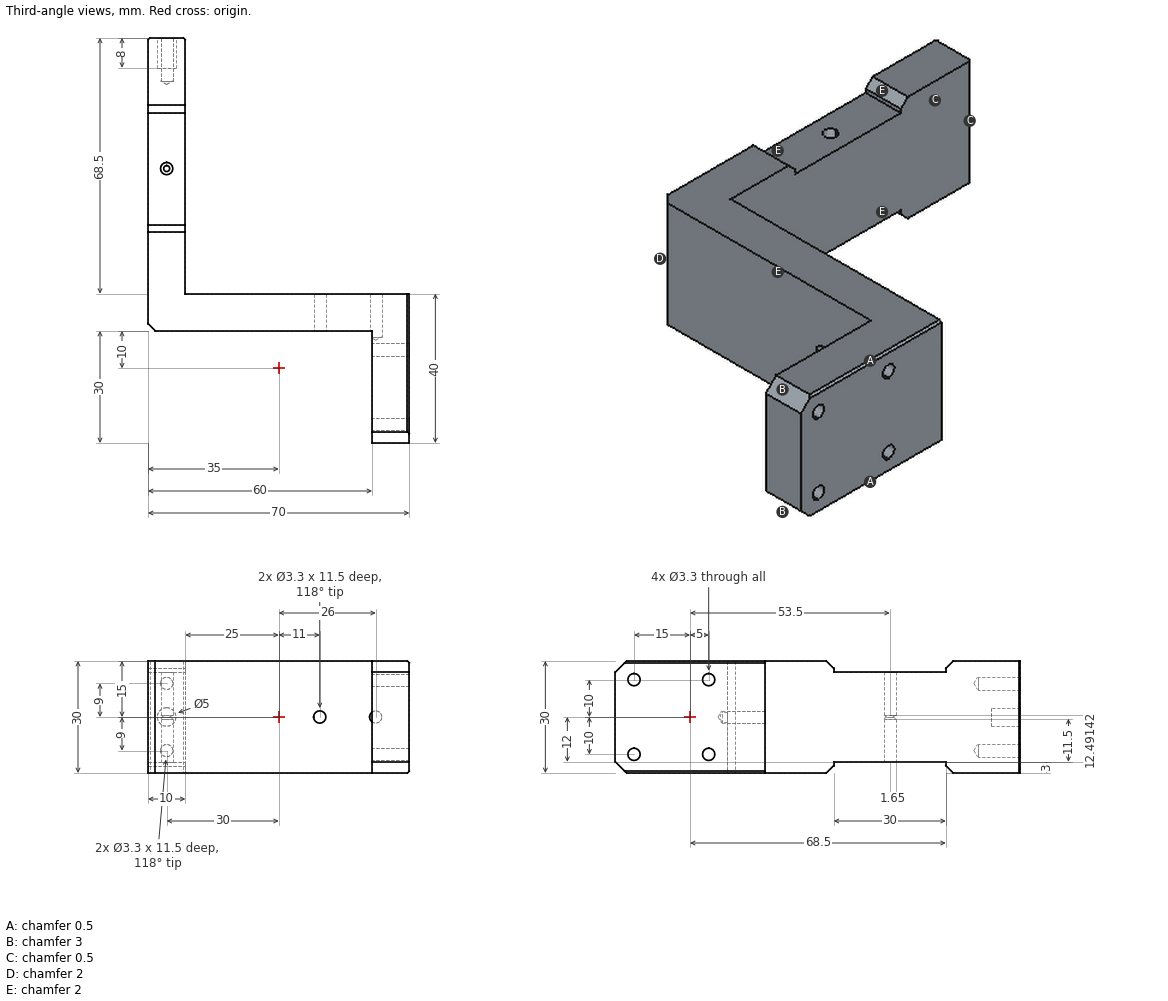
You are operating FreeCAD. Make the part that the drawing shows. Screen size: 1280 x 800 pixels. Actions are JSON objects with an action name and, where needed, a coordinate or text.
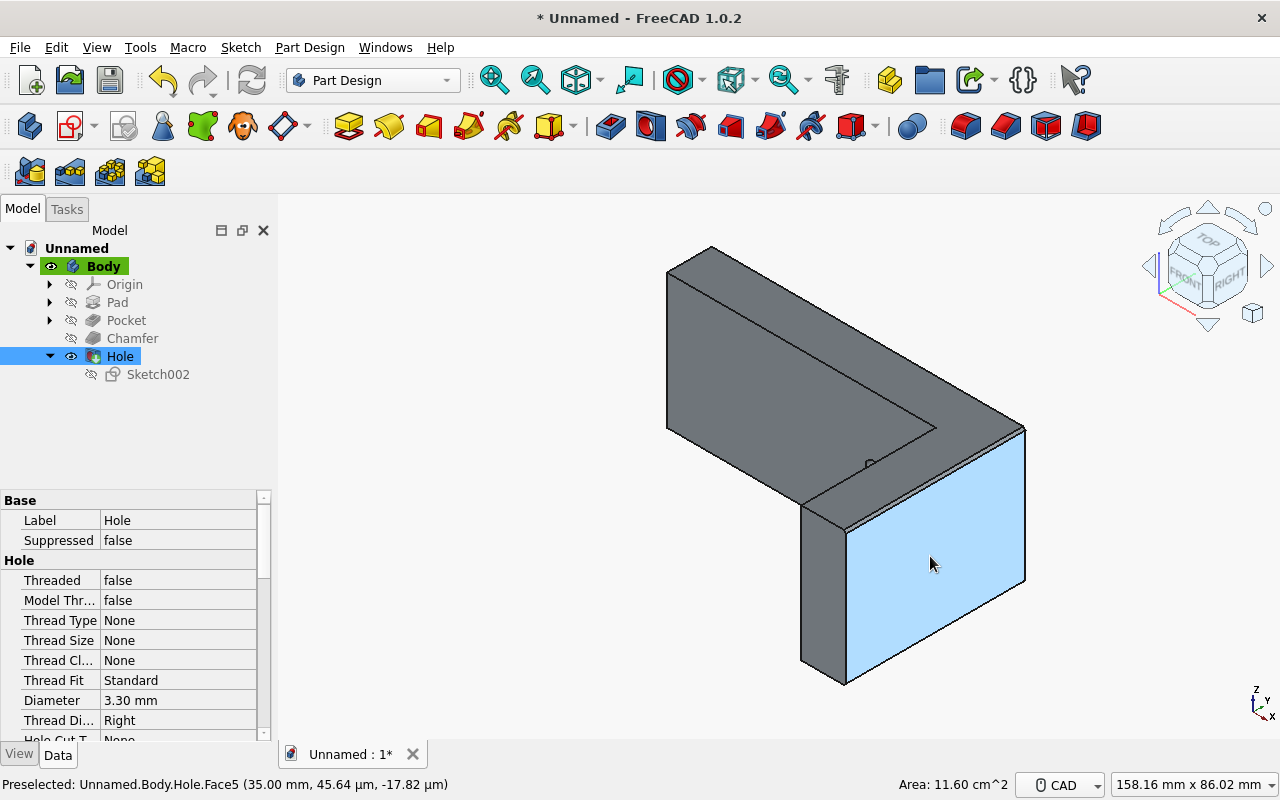
{"action": "left_click", "coordinate": [70, 126]}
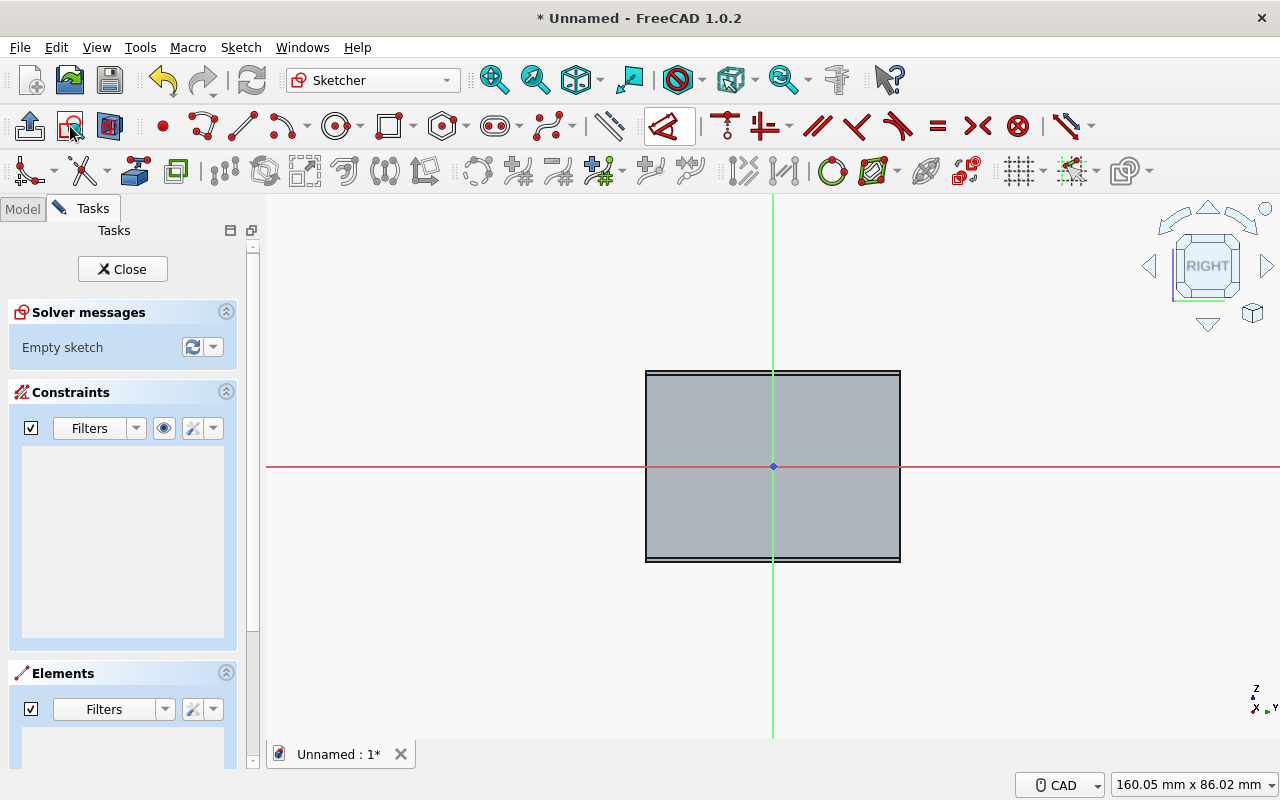
{"action": "scroll", "coordinate": [771, 466], "scroll_direction": "up", "scroll_amount": 4}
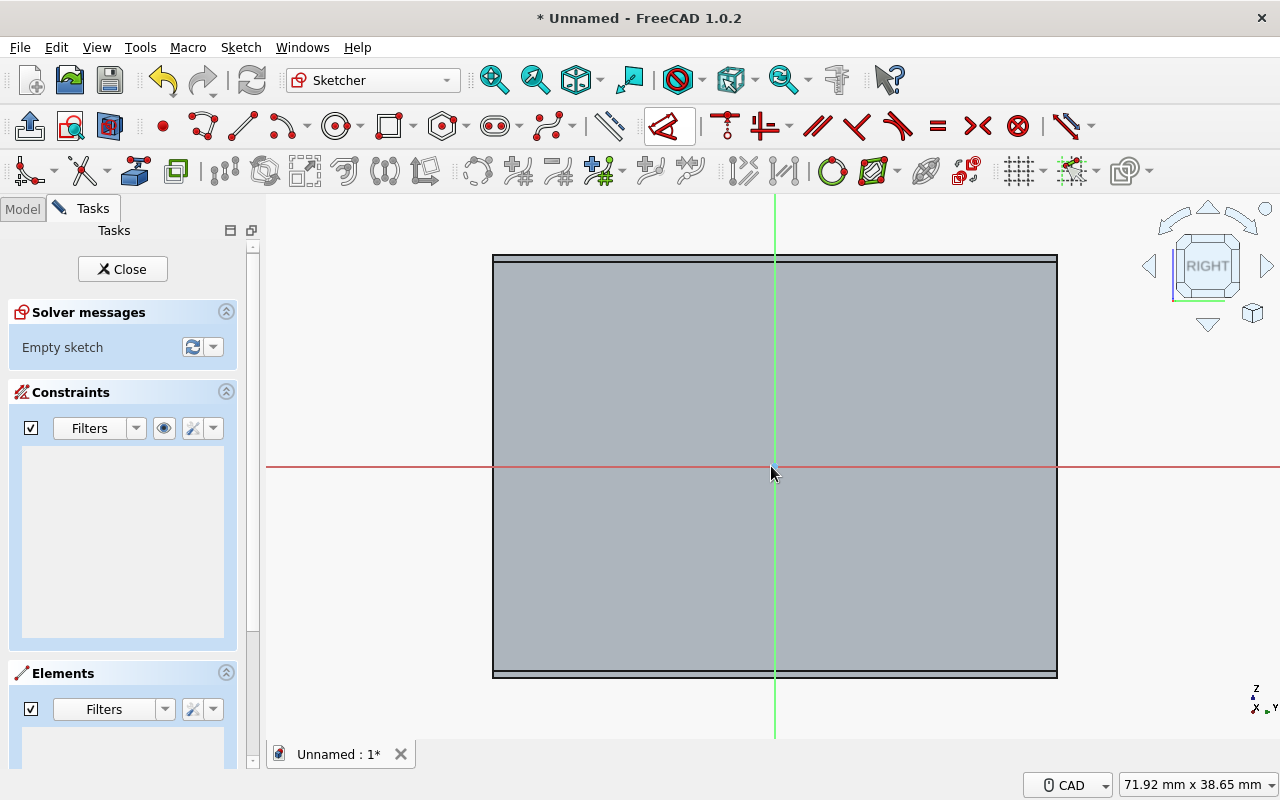
{"action": "left_click", "coordinate": [336, 126]}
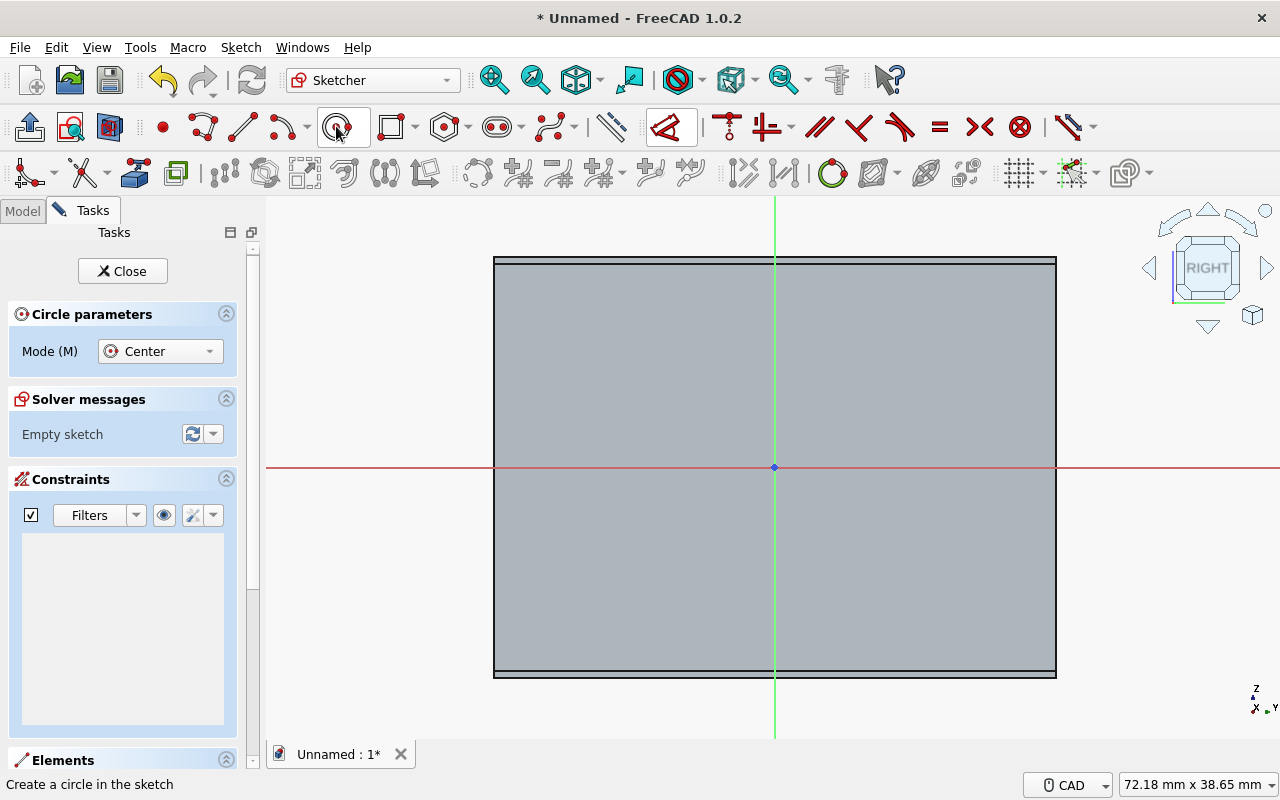
{"action": "left_click", "coordinate": [845, 327]}
{"action": "left_click", "coordinate": [861, 311]}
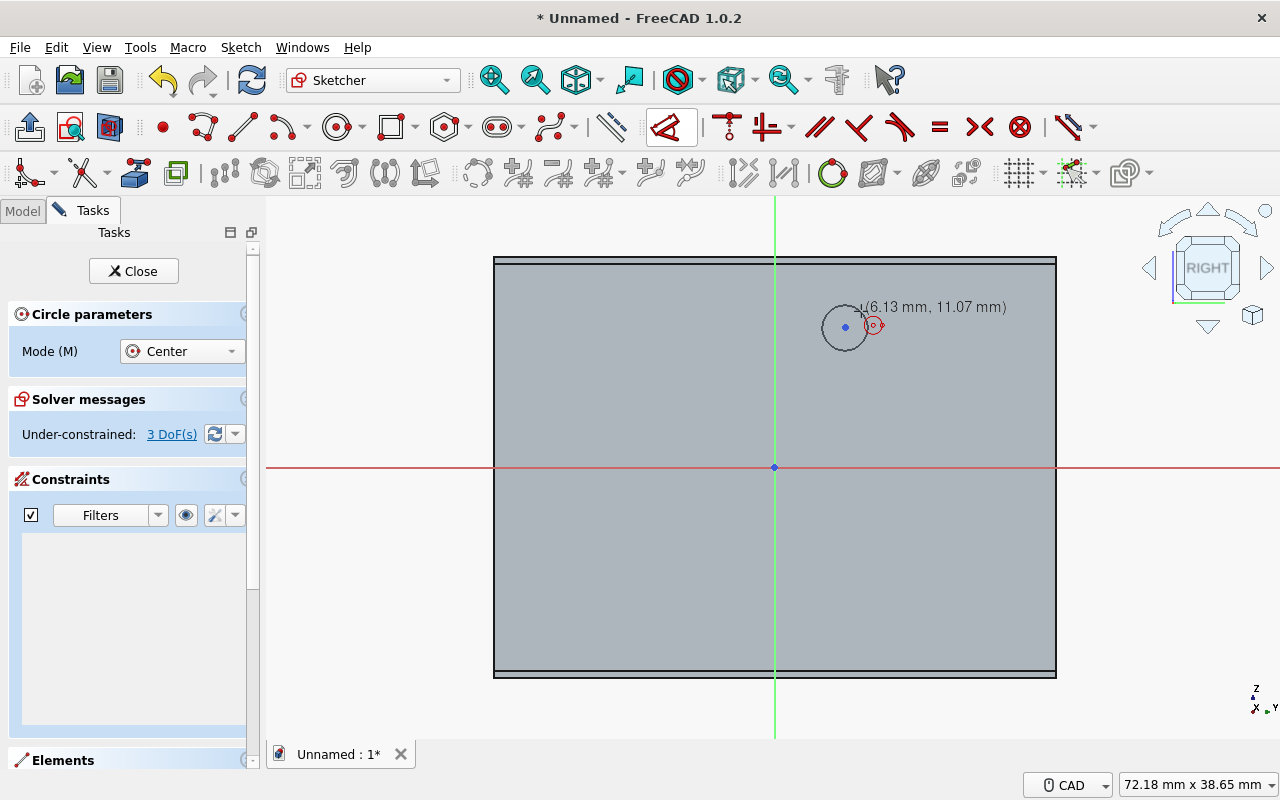
{"action": "left_click", "coordinate": [564, 327]}
{"action": "left_click", "coordinate": [581, 311]}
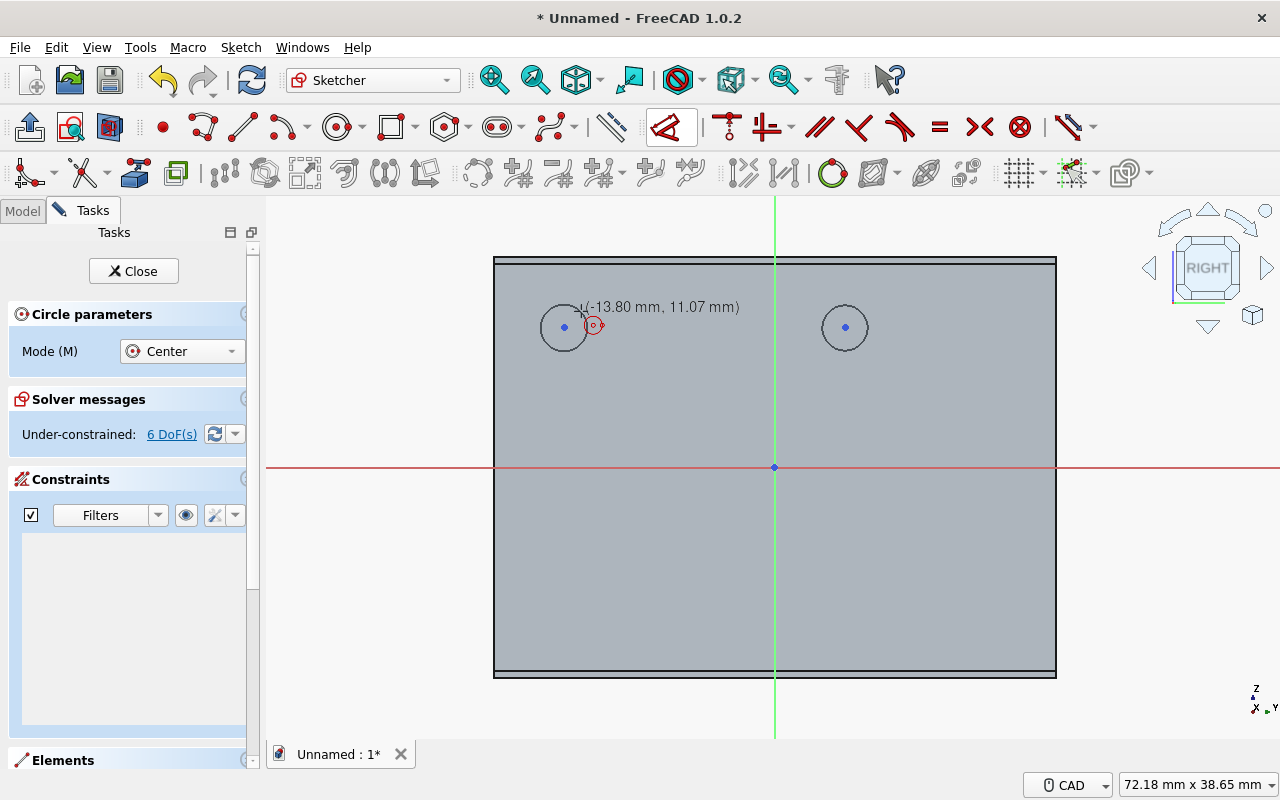
{"action": "left_click", "coordinate": [564, 608]}
{"action": "left_click", "coordinate": [581, 592]}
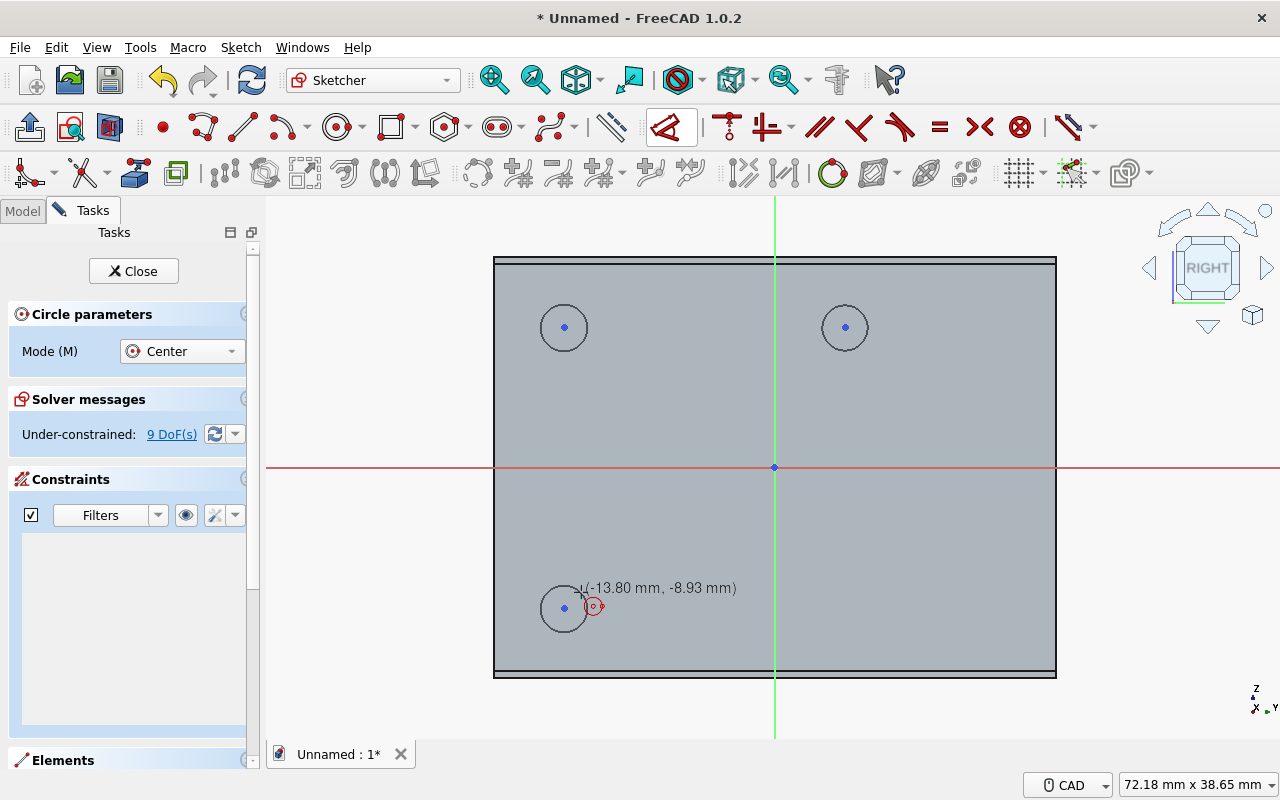
{"action": "left_click", "coordinate": [845, 608]}
{"action": "left_click", "coordinate": [861, 592]}
{"action": "key", "text": "Escape"}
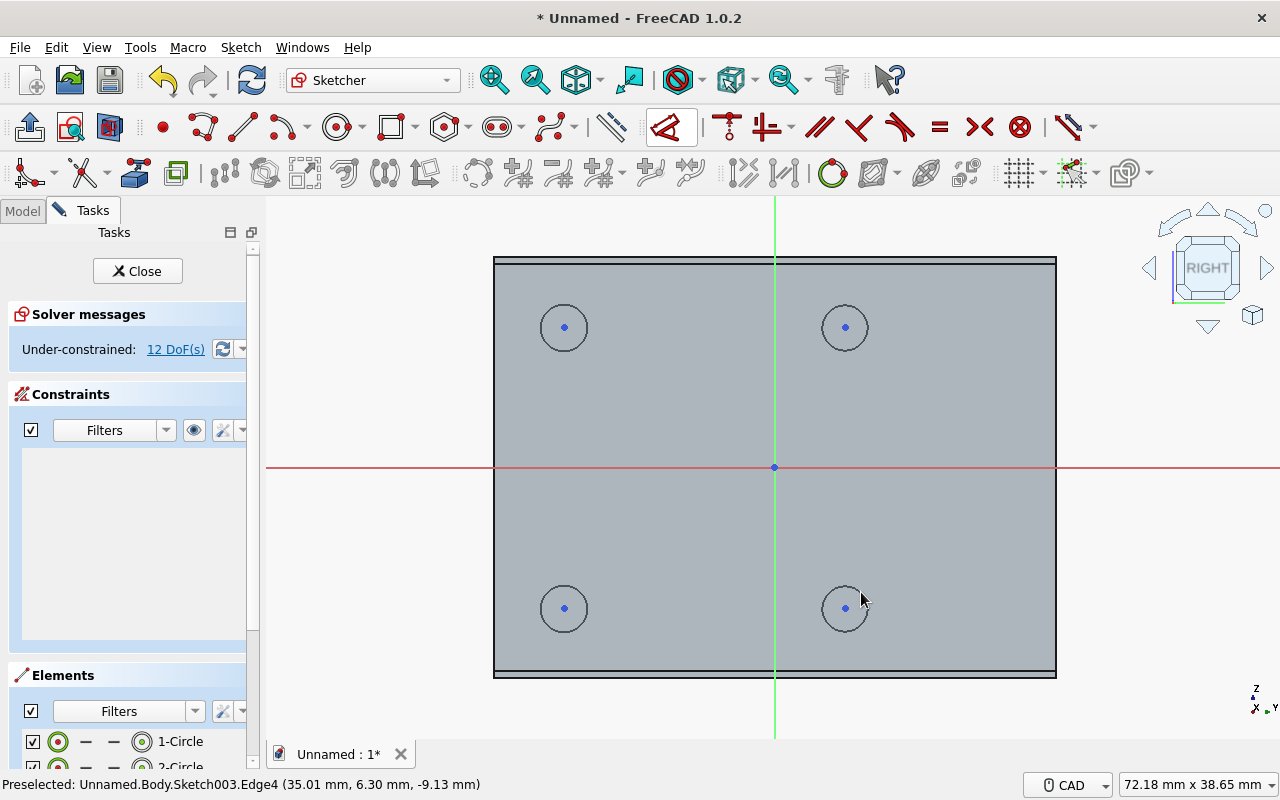
{"action": "left_click", "coordinate": [861, 312]}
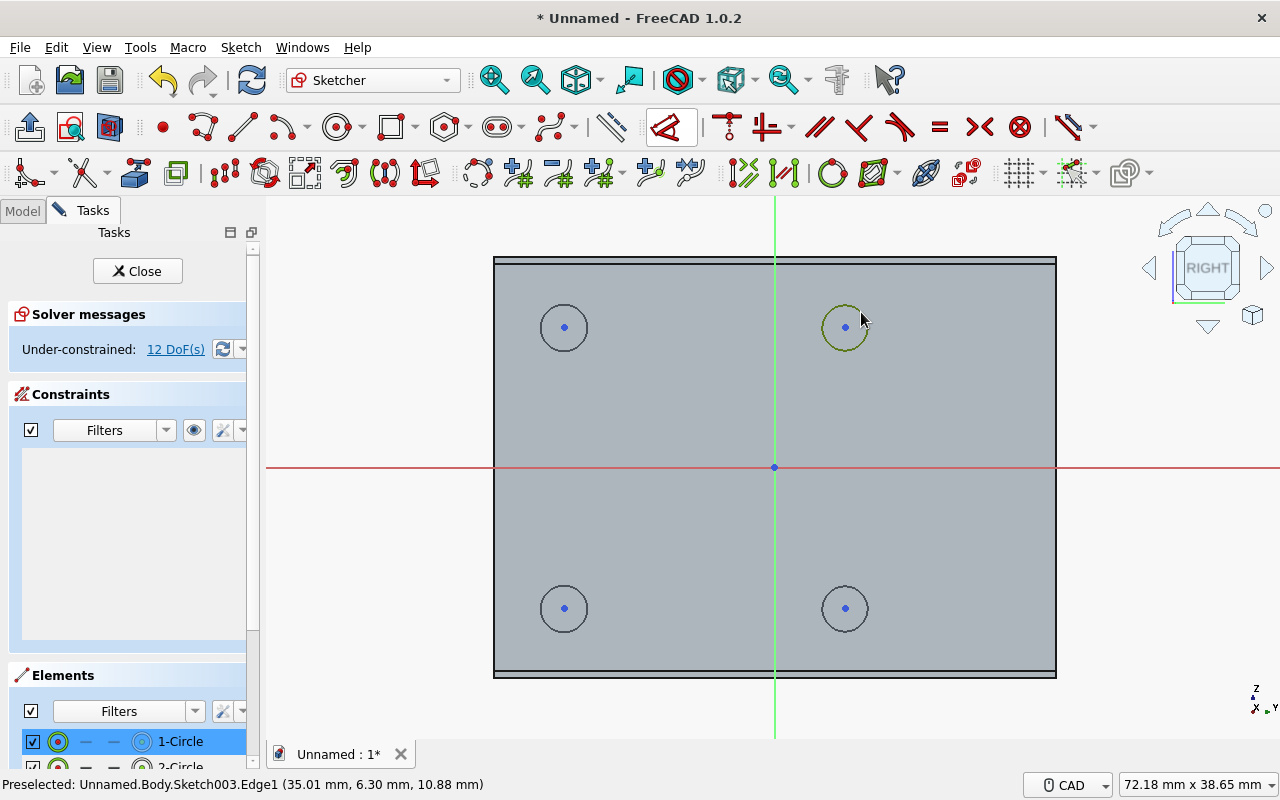
{"action": "left_click", "coordinate": [580, 311]}